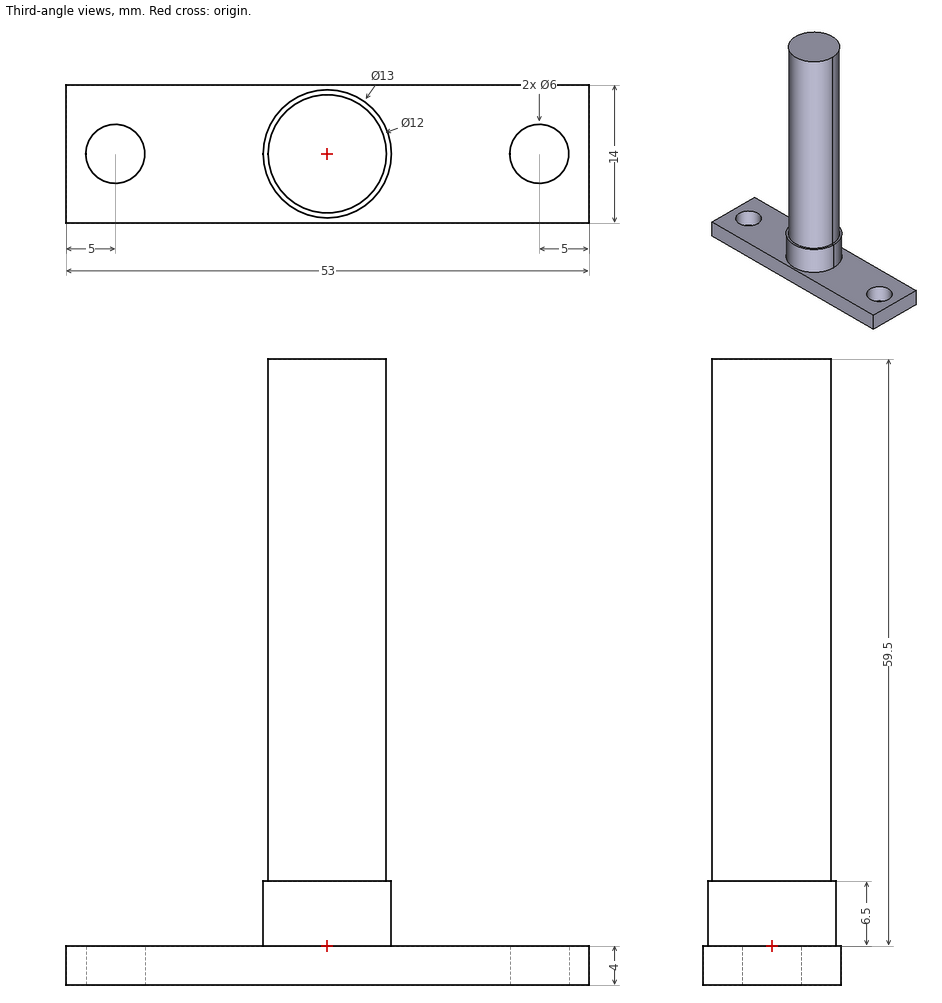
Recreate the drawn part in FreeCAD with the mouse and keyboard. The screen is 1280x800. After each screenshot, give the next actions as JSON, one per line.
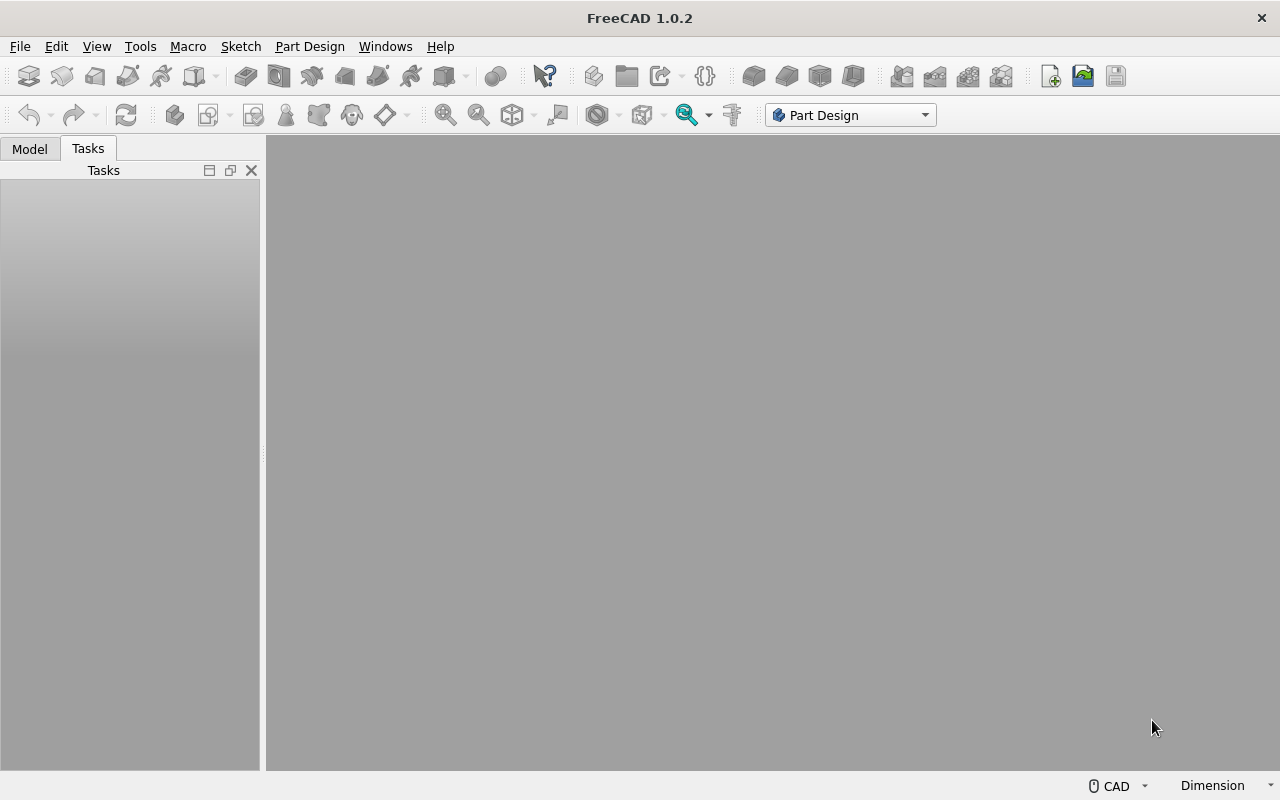
{"action": "key", "text": "ctrl+n"}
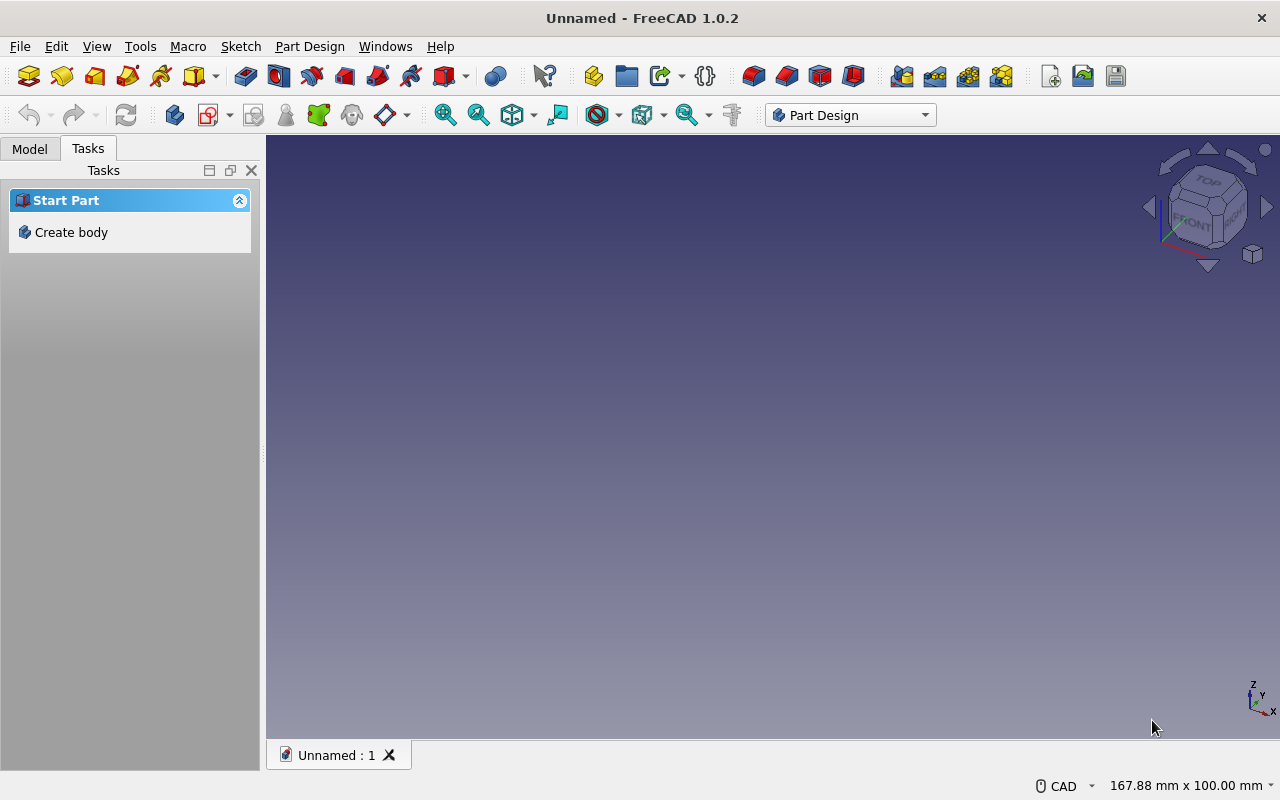
{"action": "left_click", "coordinate": [208, 116]}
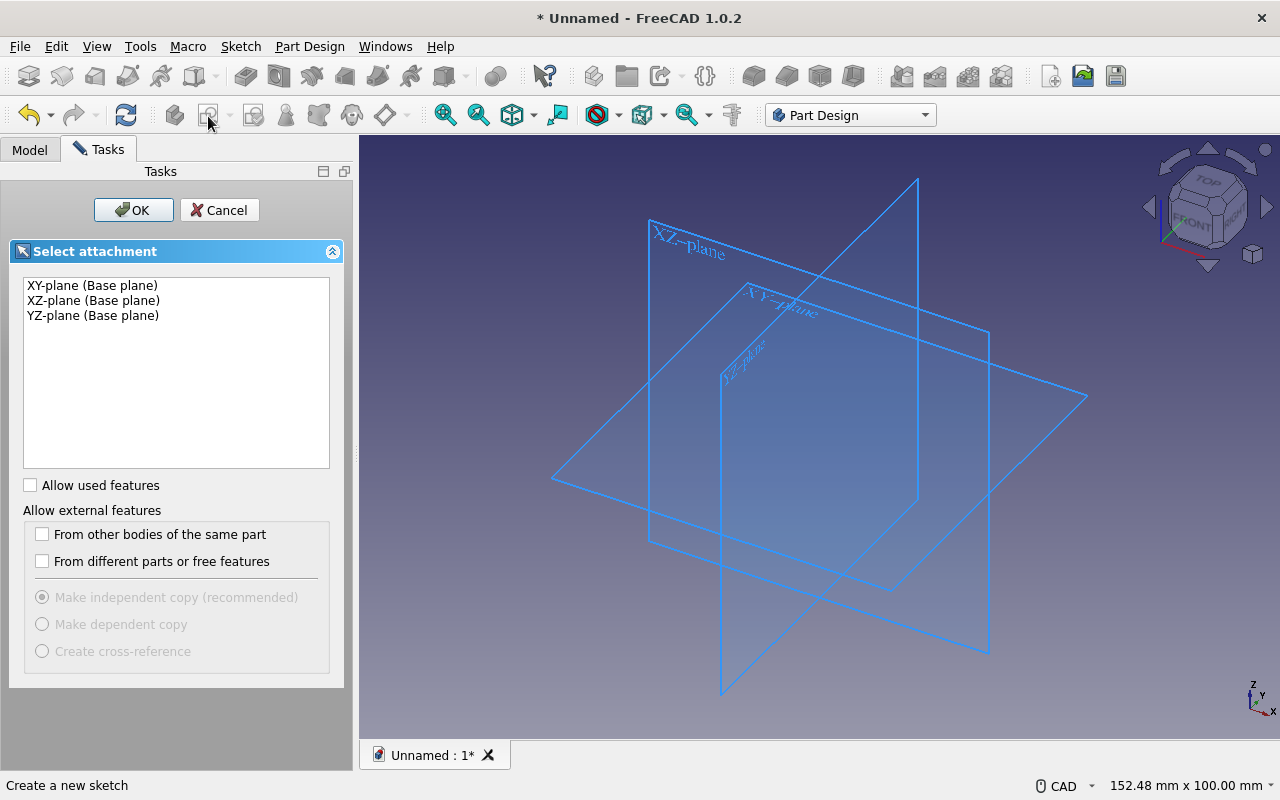
{"action": "left_click", "coordinate": [84, 286]}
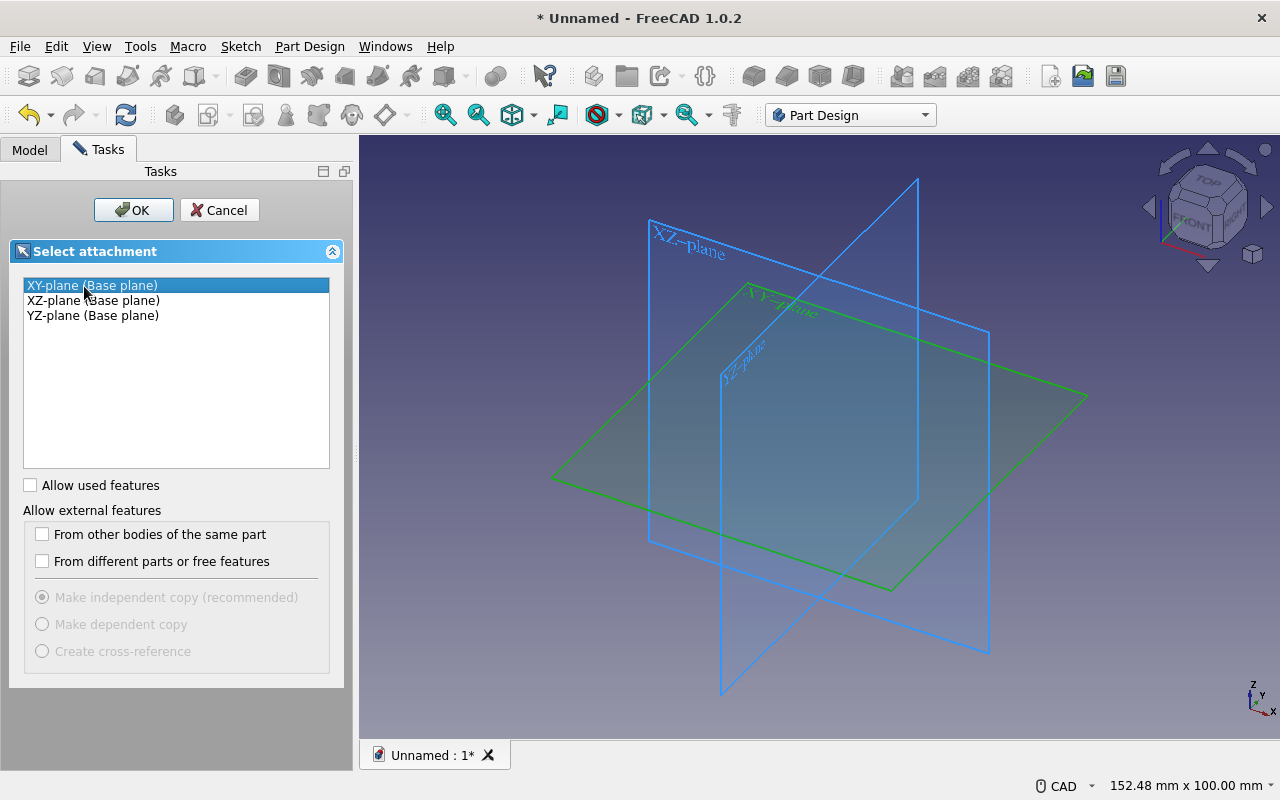
{"action": "left_click", "coordinate": [134, 210]}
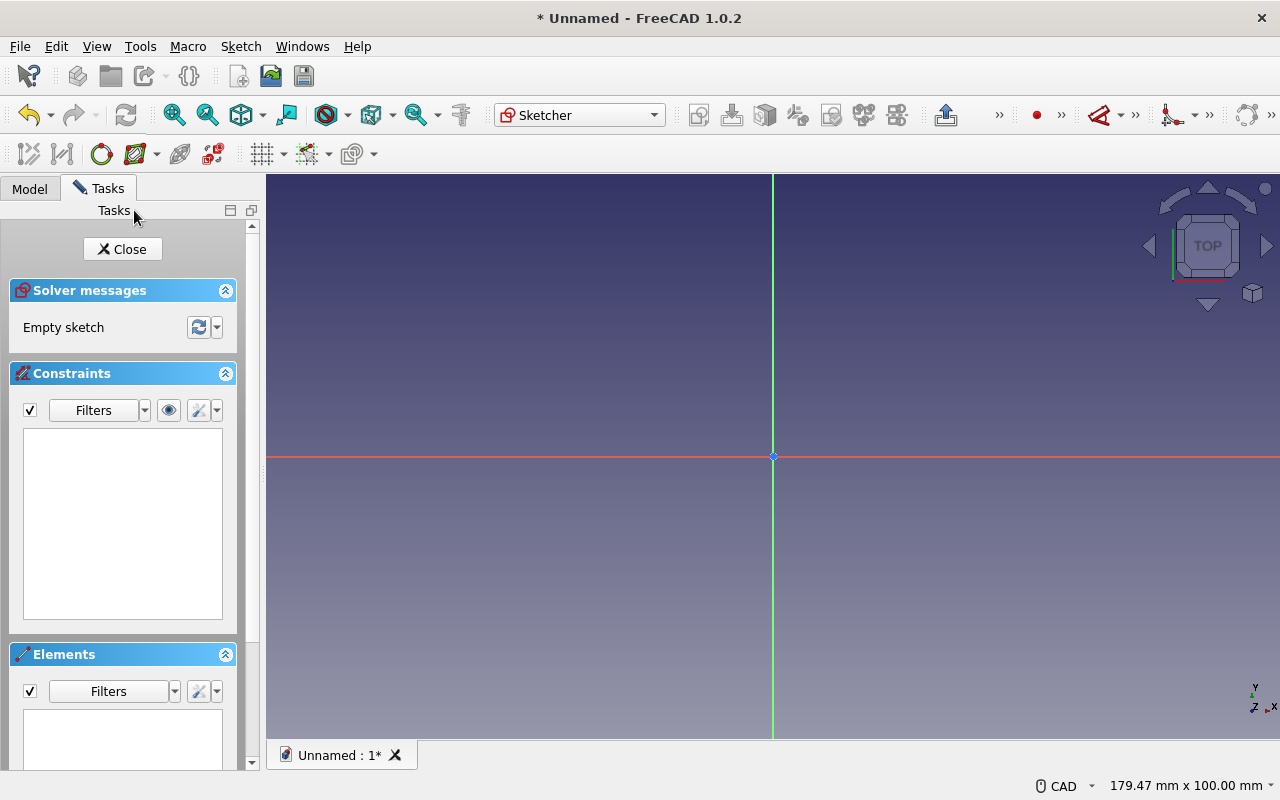
{"action": "scroll", "coordinate": [790, 456], "scroll_direction": "up", "scroll_amount": 8}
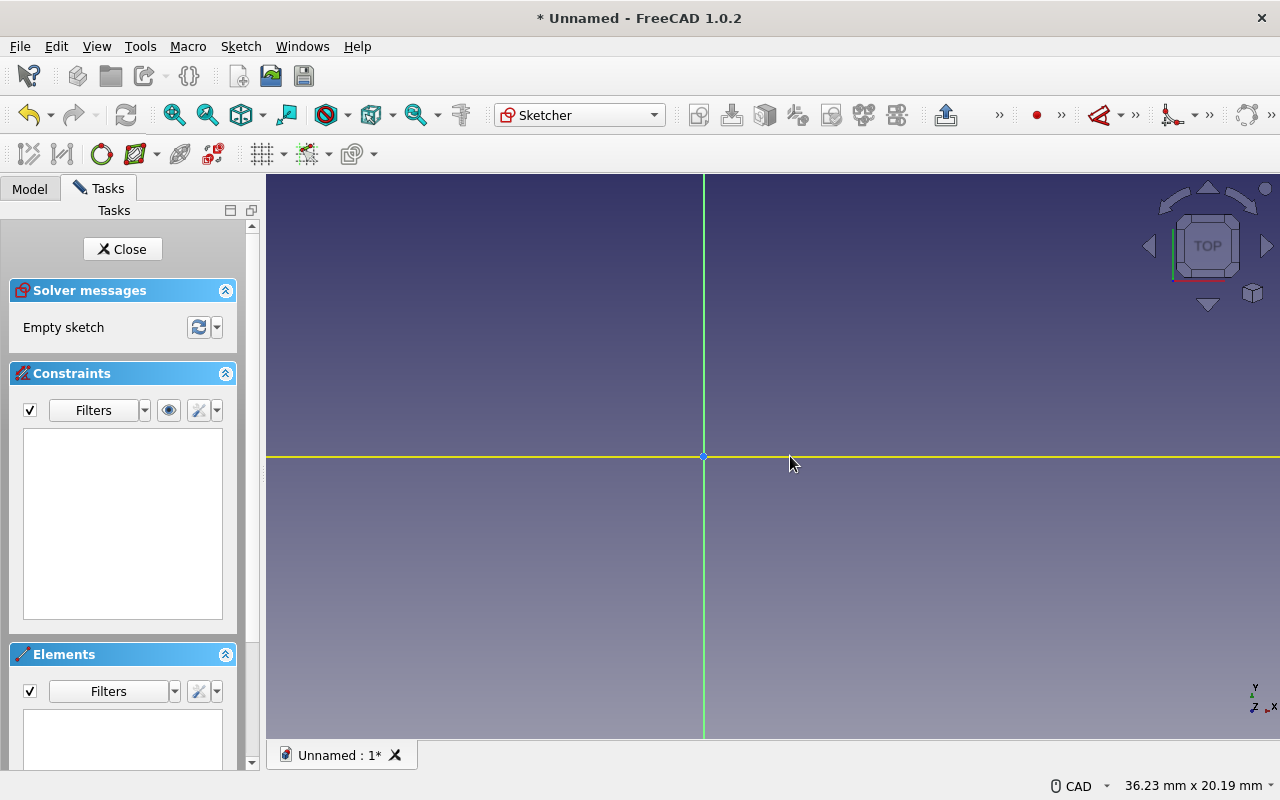
{"action": "key", "text": "g c"}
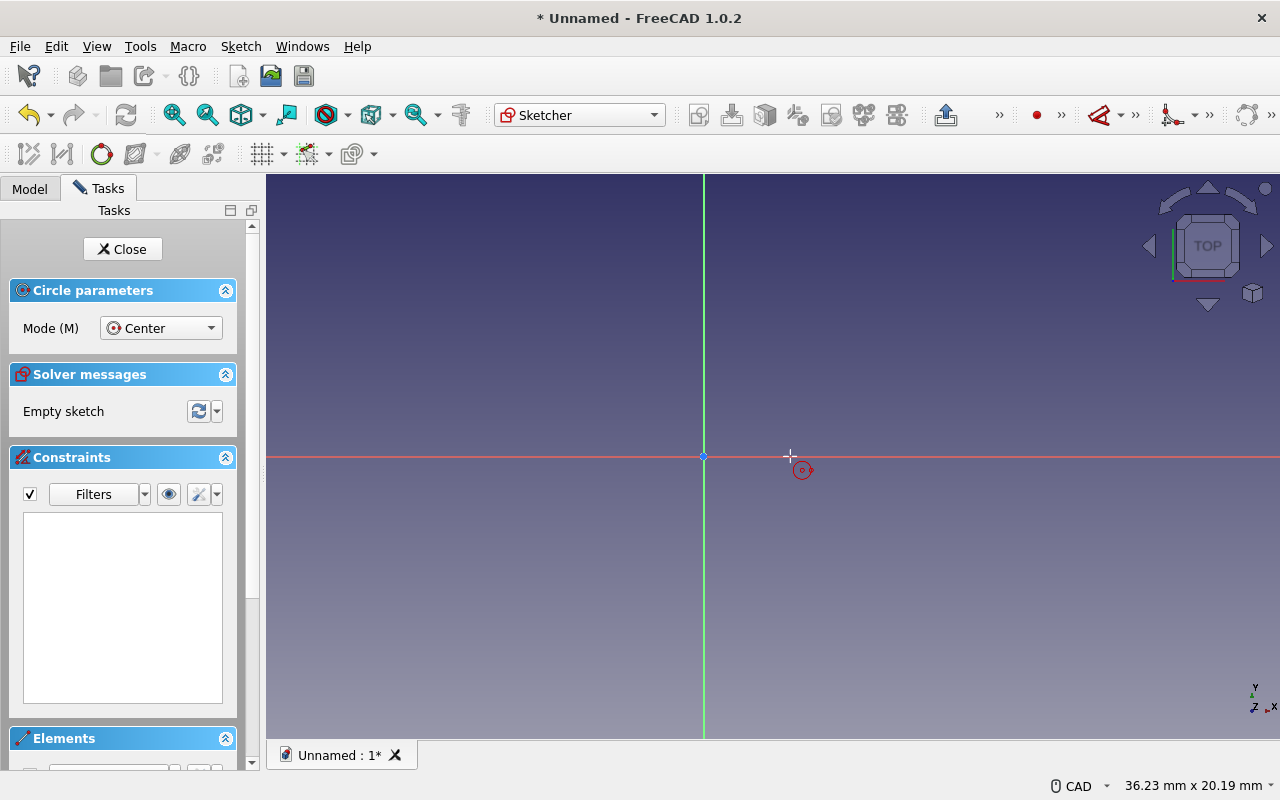
{"action": "left_click", "coordinate": [704, 456]}
{"action": "left_click", "coordinate": [822, 338]}
{"action": "key", "text": "Escape"}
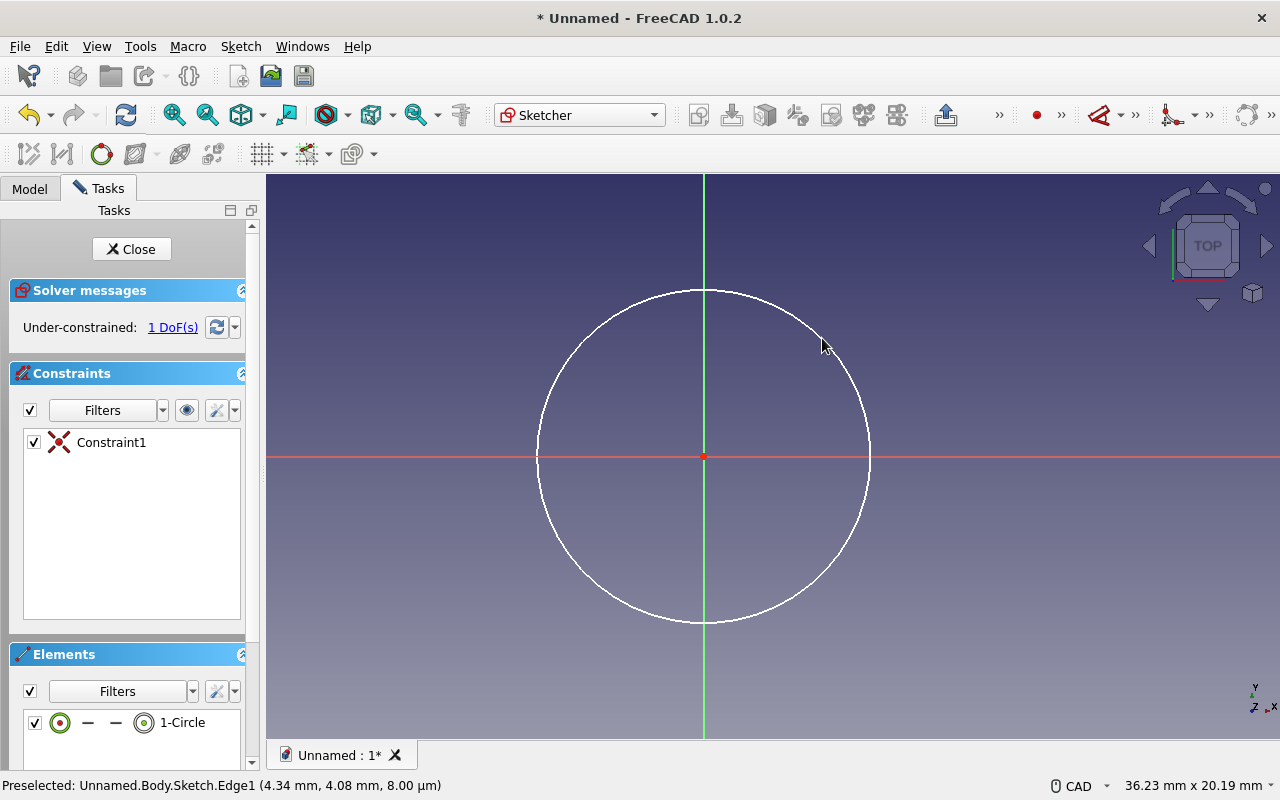
{"action": "key", "text": "d"}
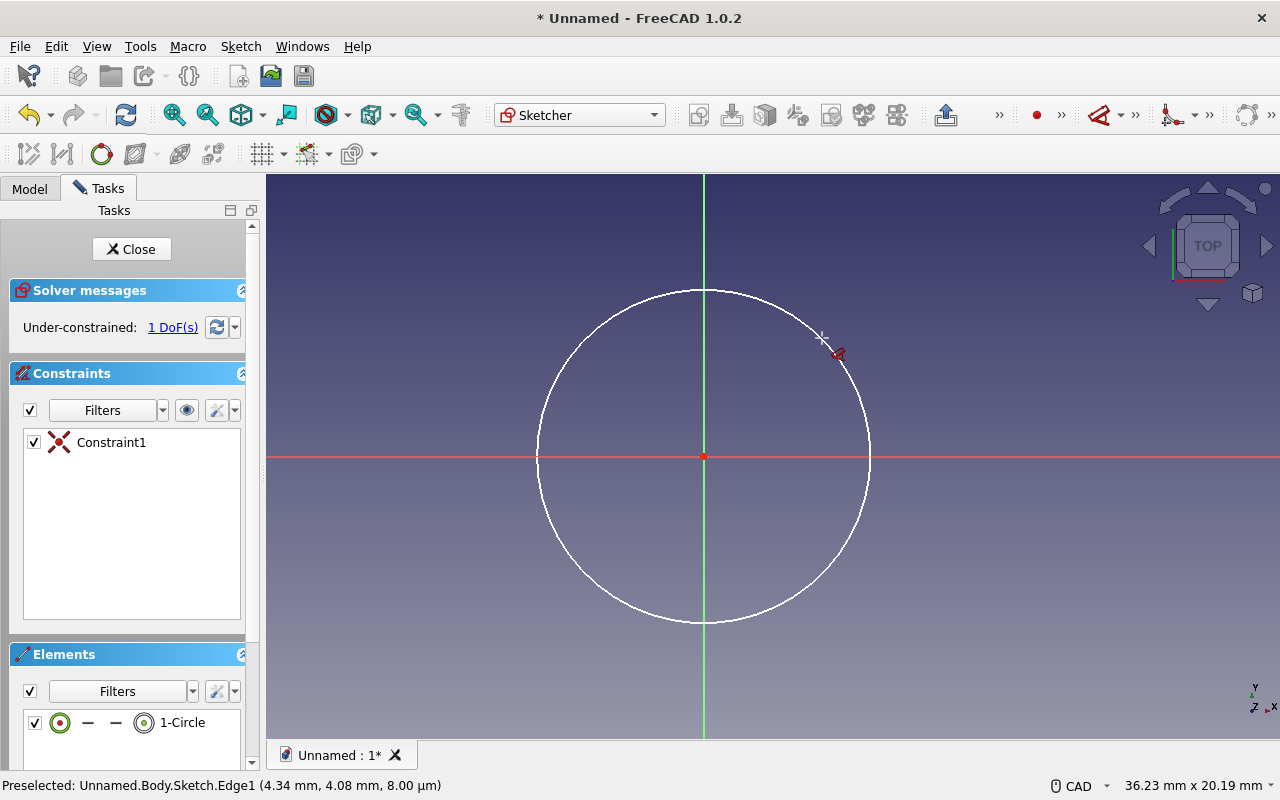
{"action": "left_click", "coordinate": [821, 338]}
{"action": "left_click", "coordinate": [844, 315]}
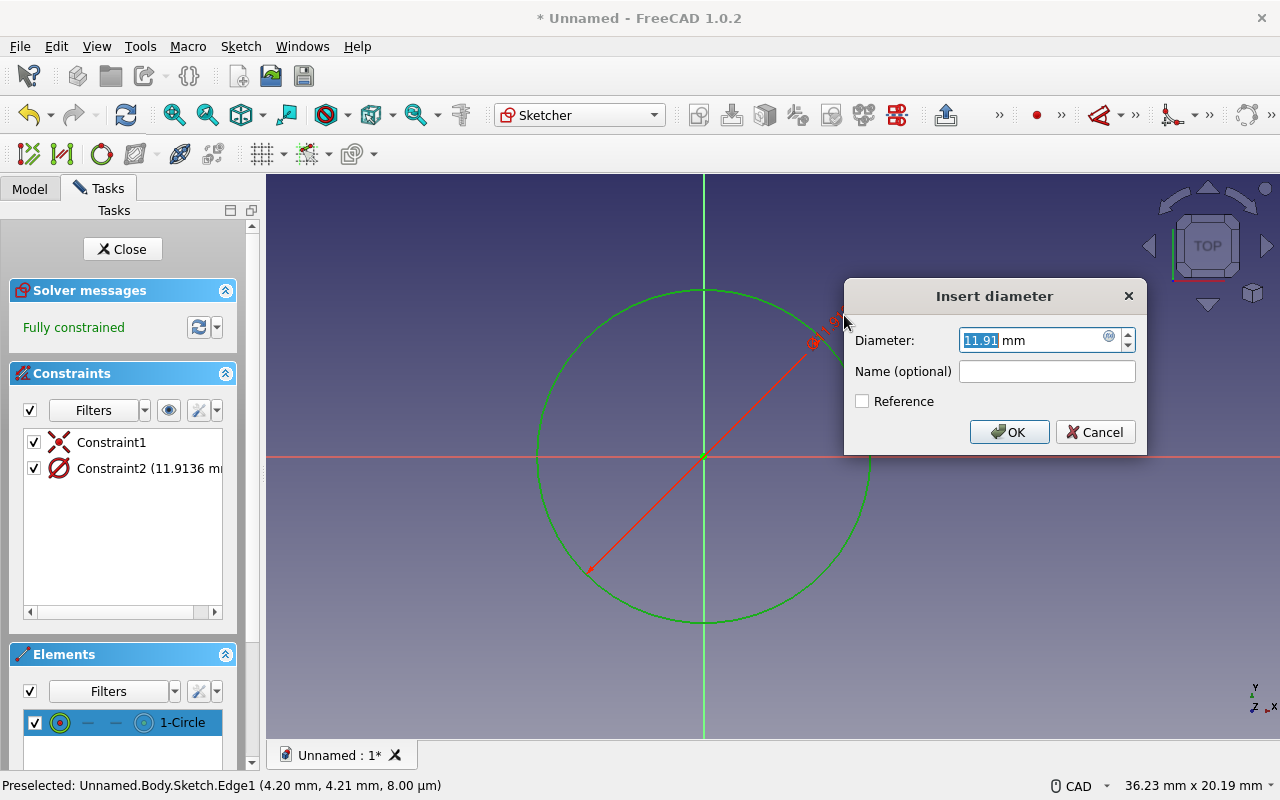
{"action": "type", "text": "12"}
{"action": "key", "text": "Return"}
{"action": "key", "text": "Escape"}